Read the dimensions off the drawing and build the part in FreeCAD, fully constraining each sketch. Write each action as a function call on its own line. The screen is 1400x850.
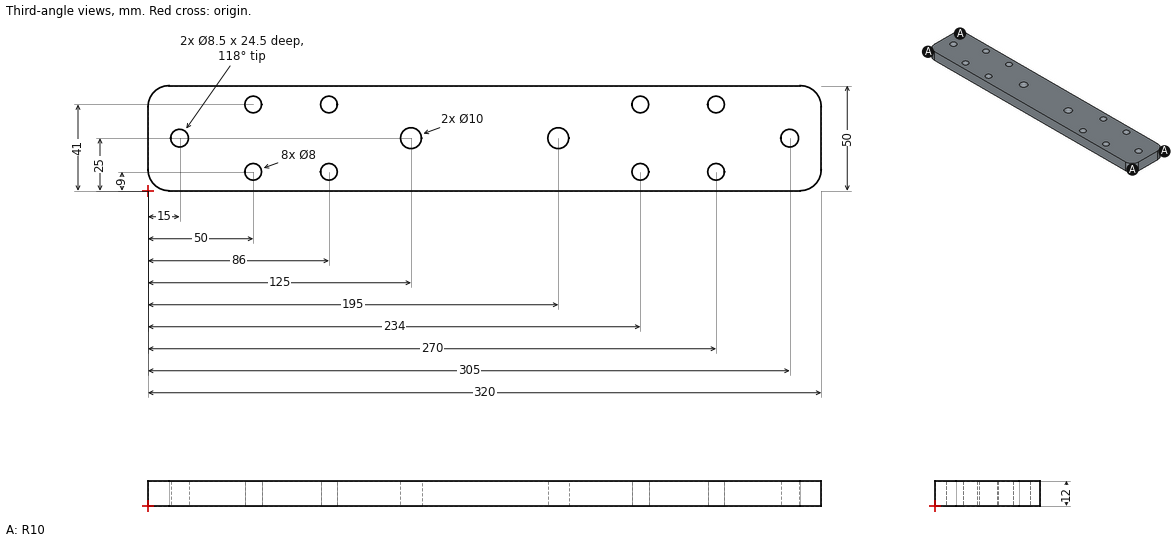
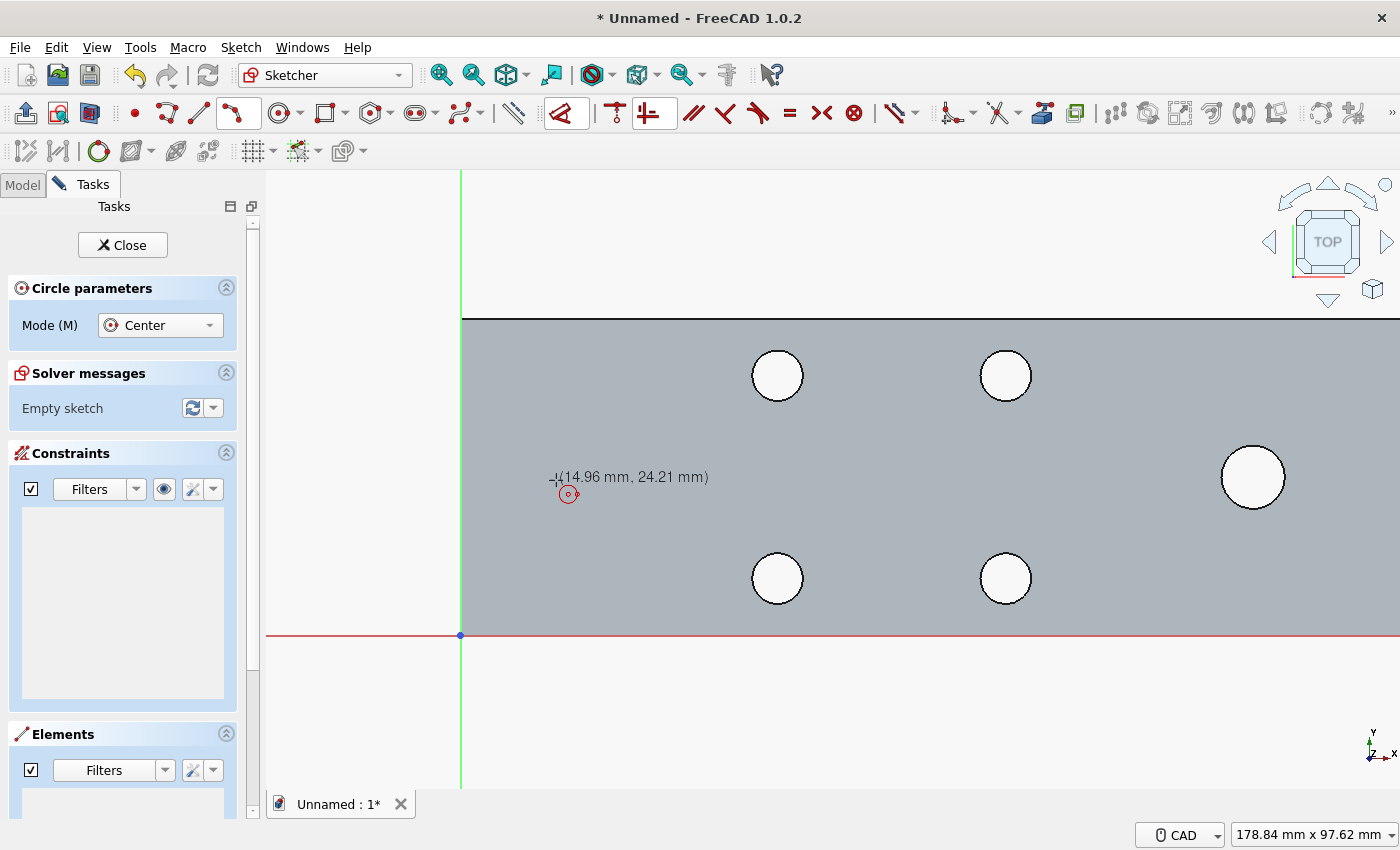
click(556, 477)
click(575, 458)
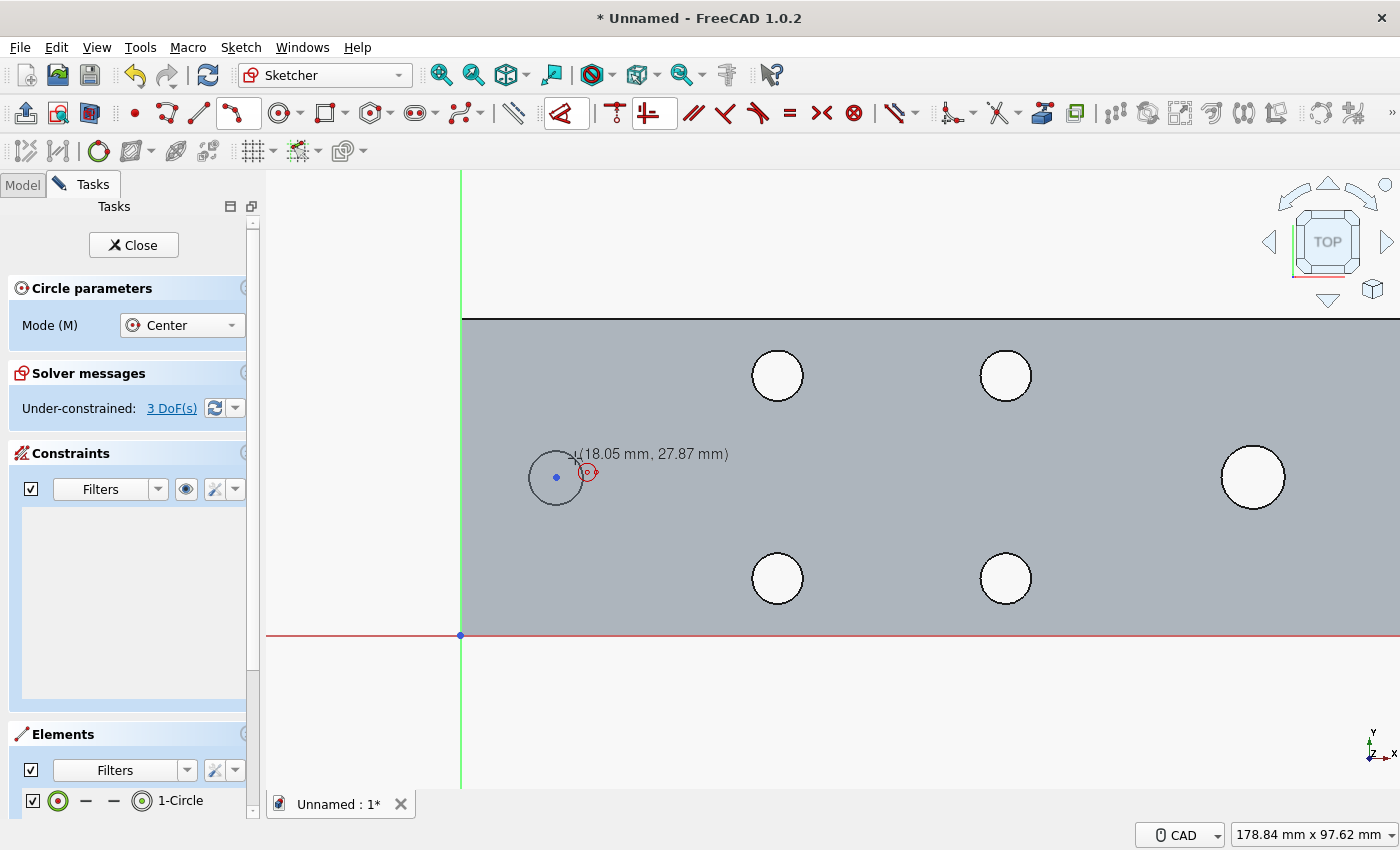
scroll(371, 443, down, 5)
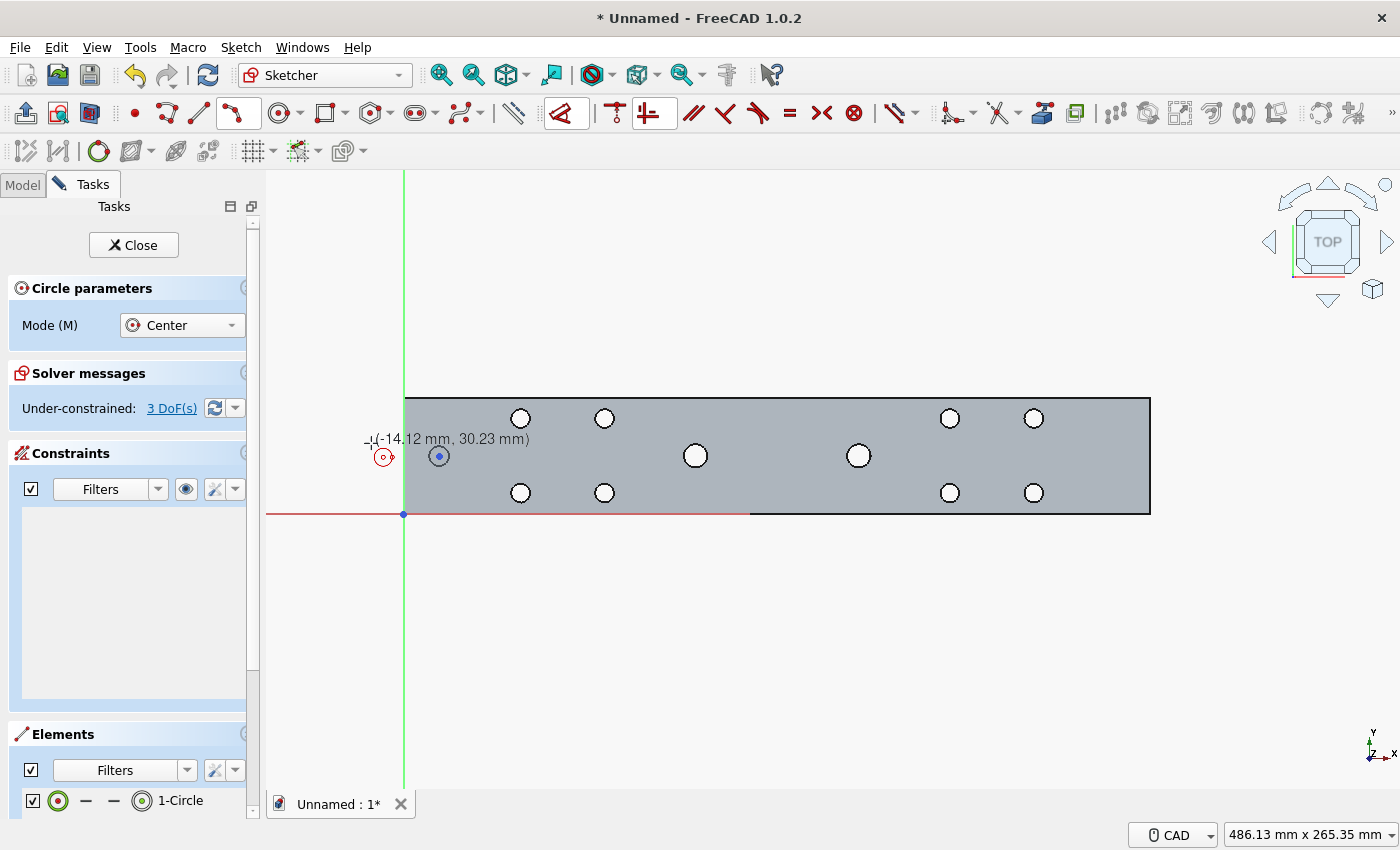
scroll(1115, 456, up, 5)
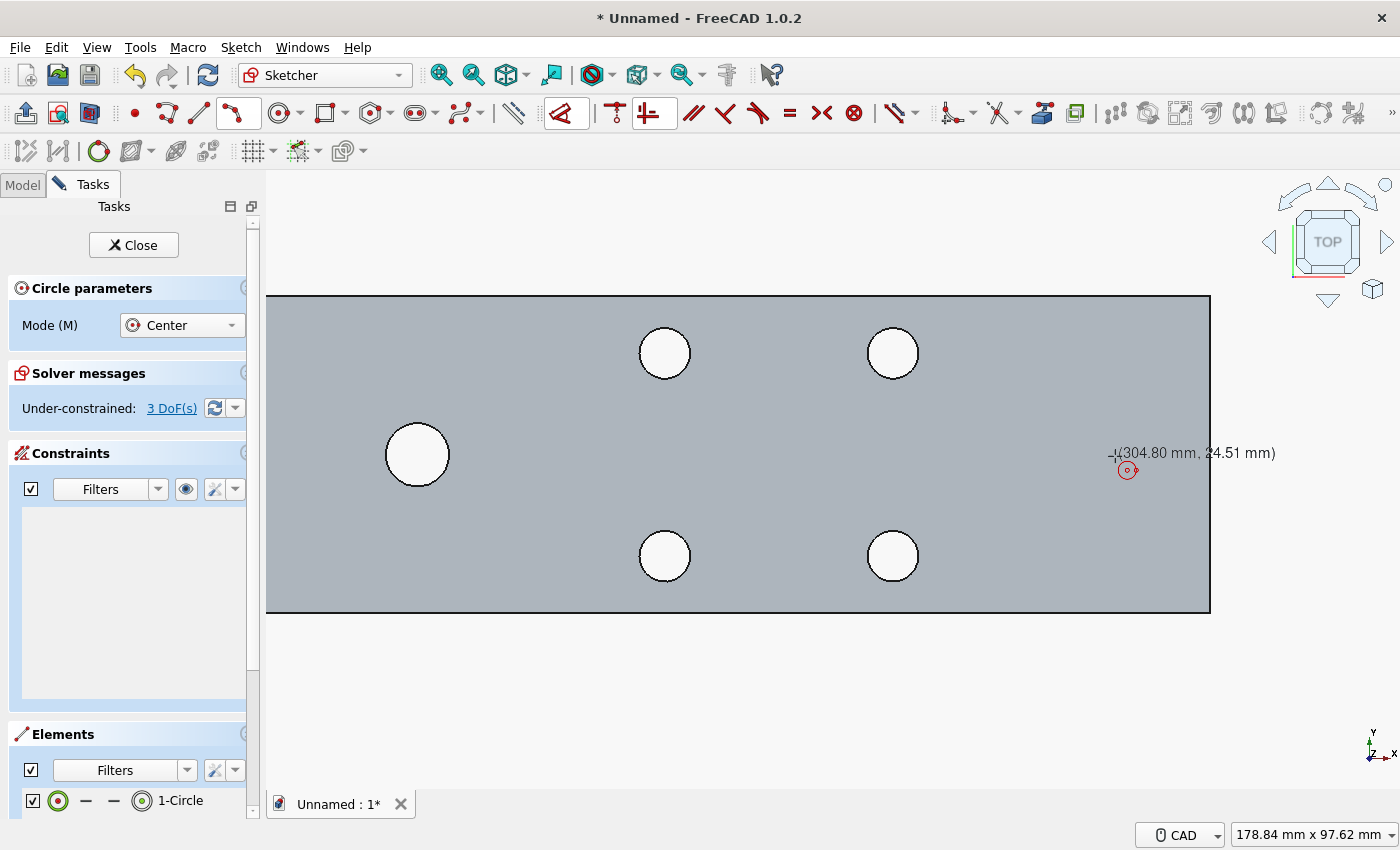
click(1115, 455)
click(1134, 436)
key(Escape)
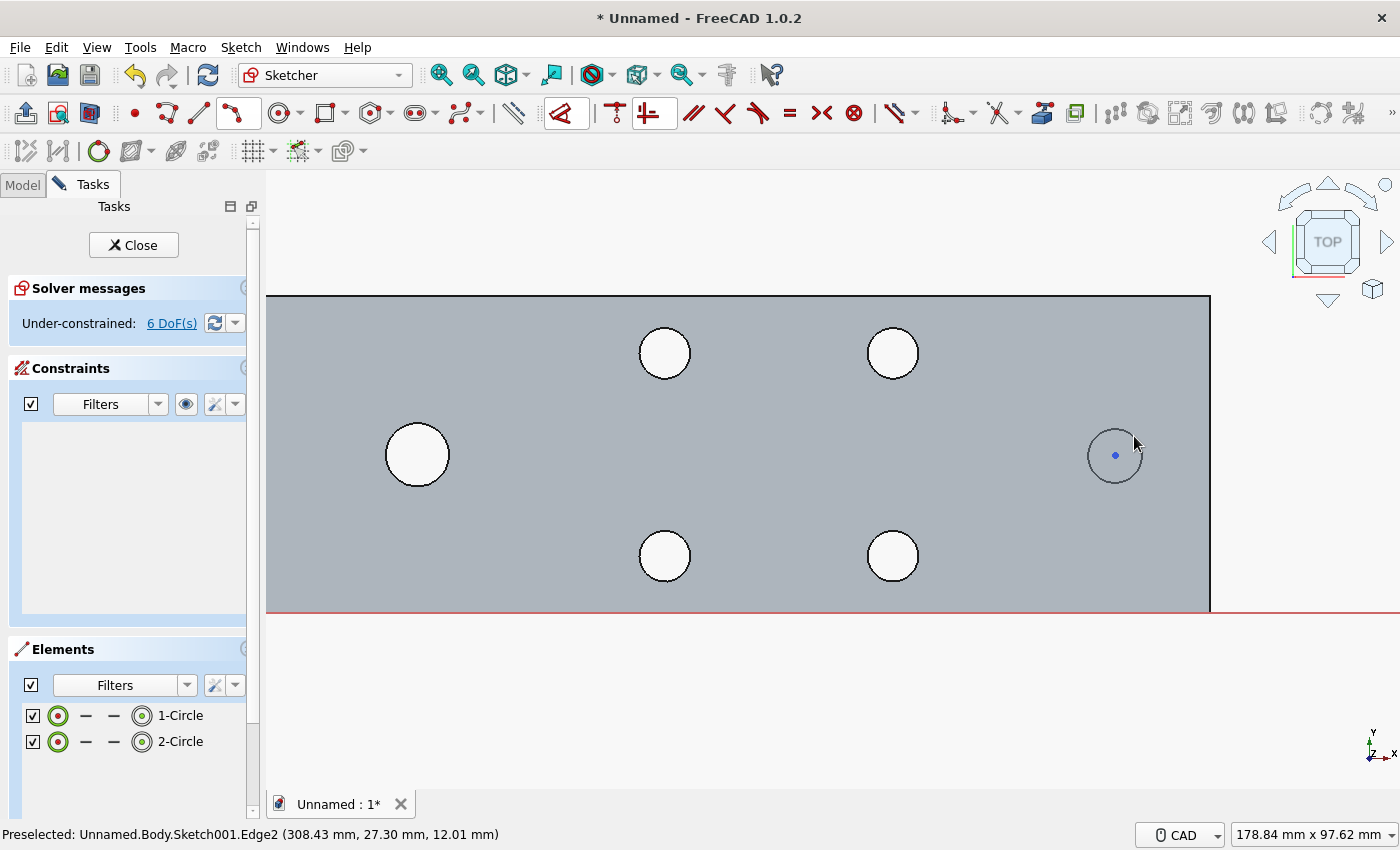
scroll(1115, 456, down, 5)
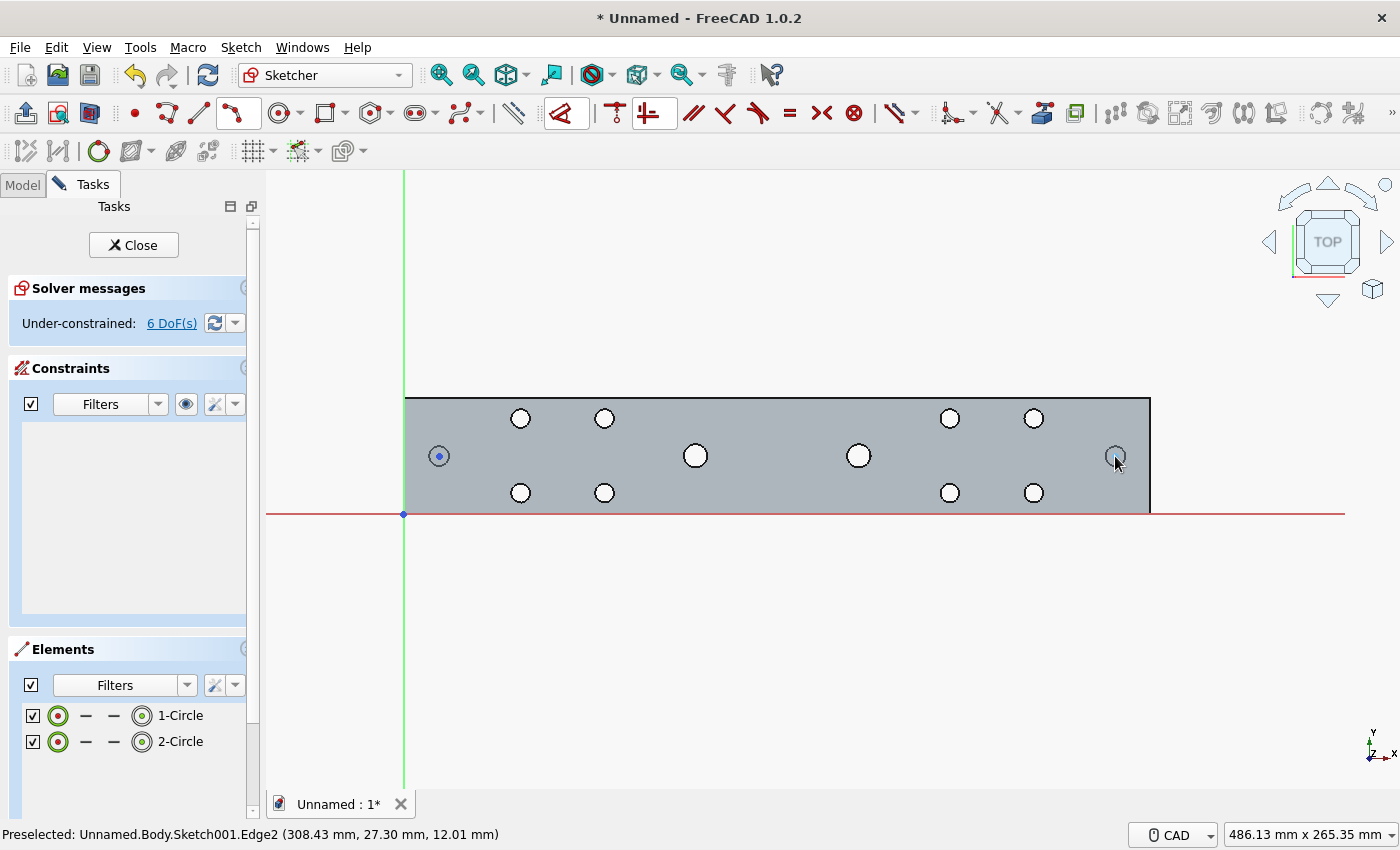
scroll(446, 449, up, 2)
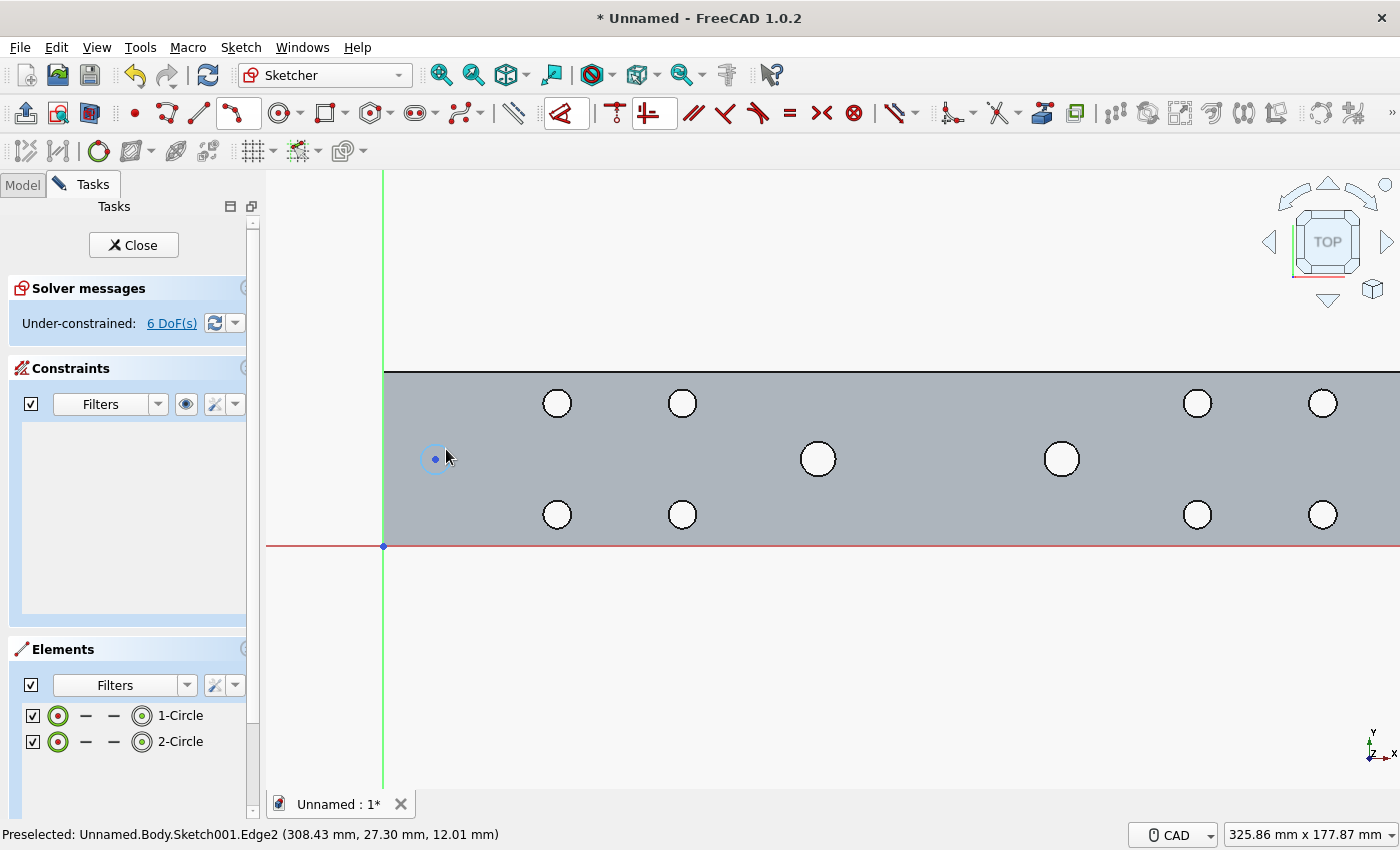
click(446, 449)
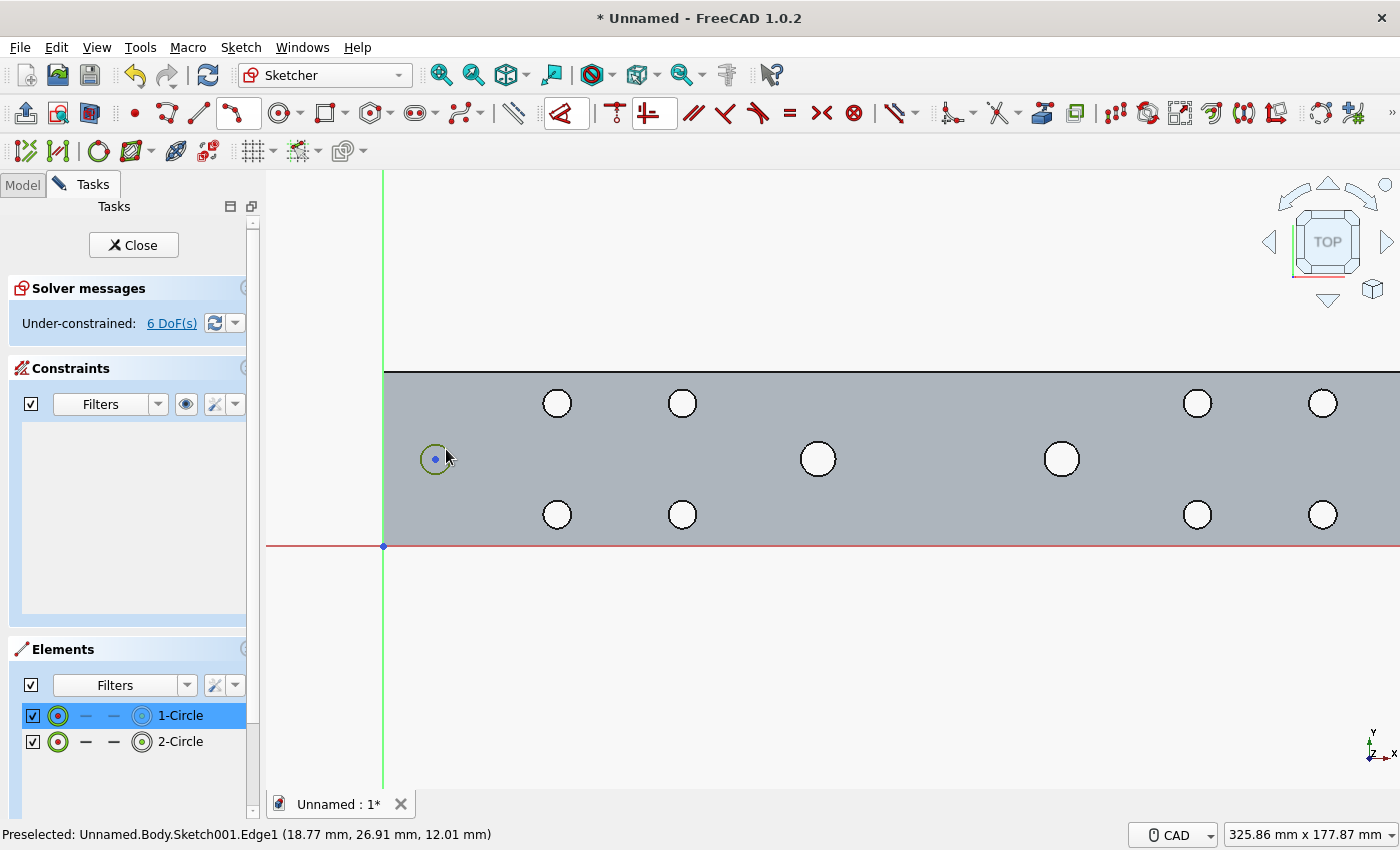
scroll(446, 448, down, 2)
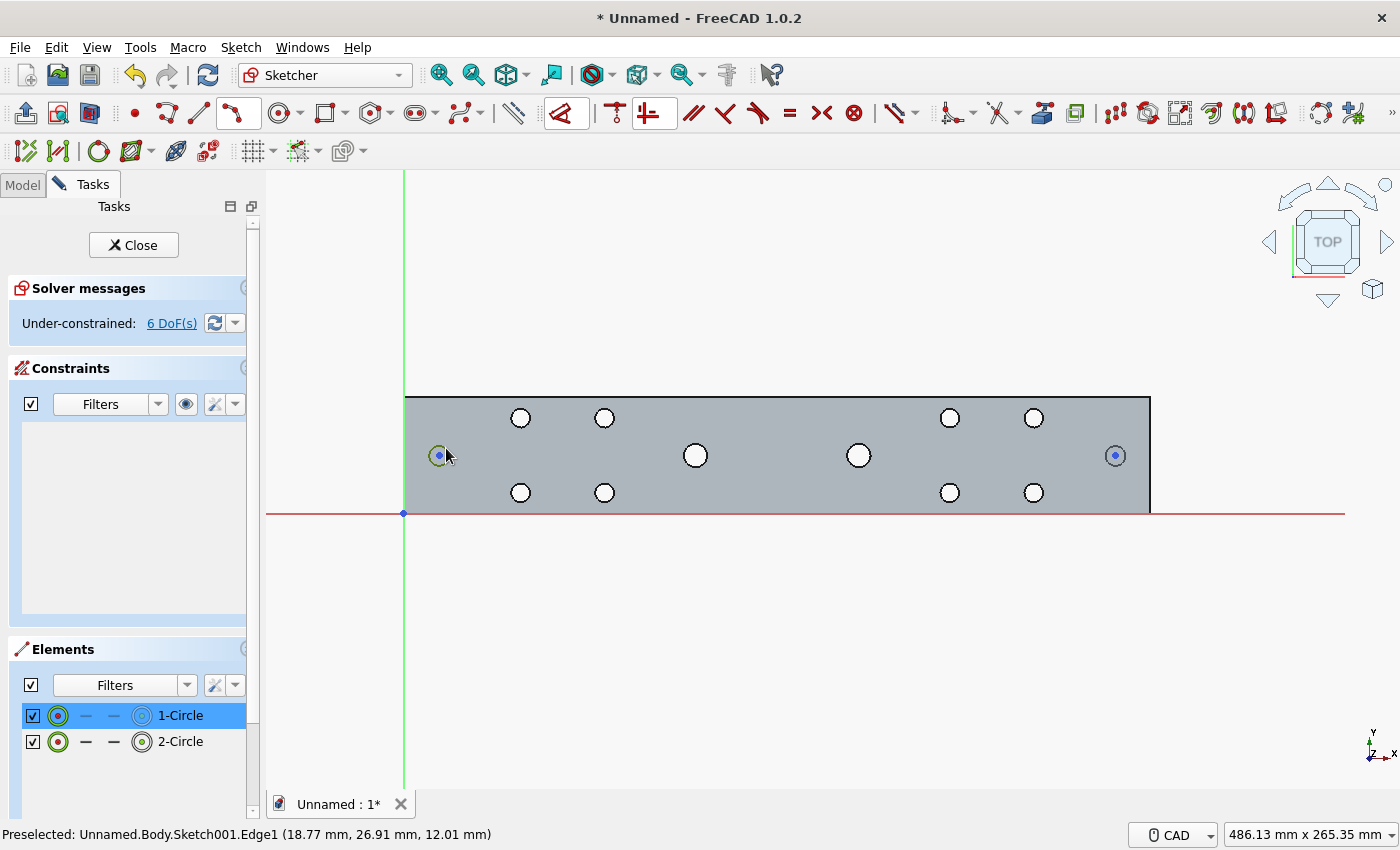
scroll(1122, 449, up, 2)